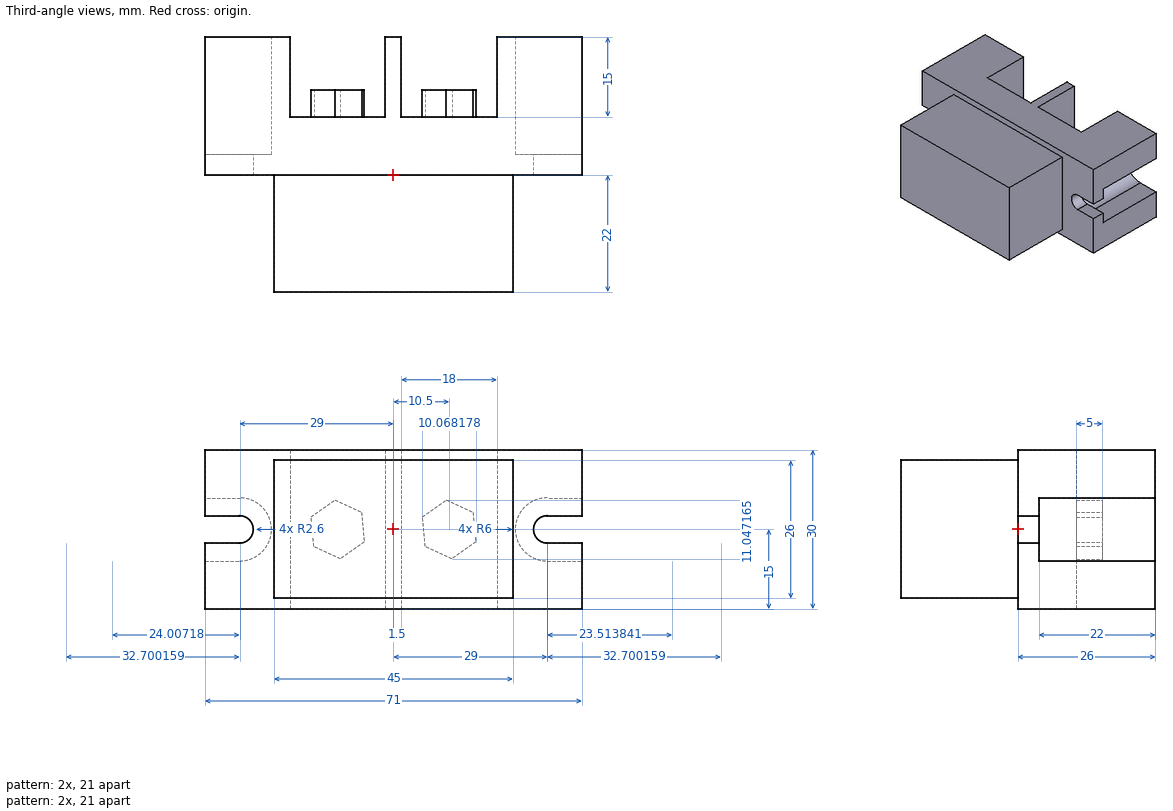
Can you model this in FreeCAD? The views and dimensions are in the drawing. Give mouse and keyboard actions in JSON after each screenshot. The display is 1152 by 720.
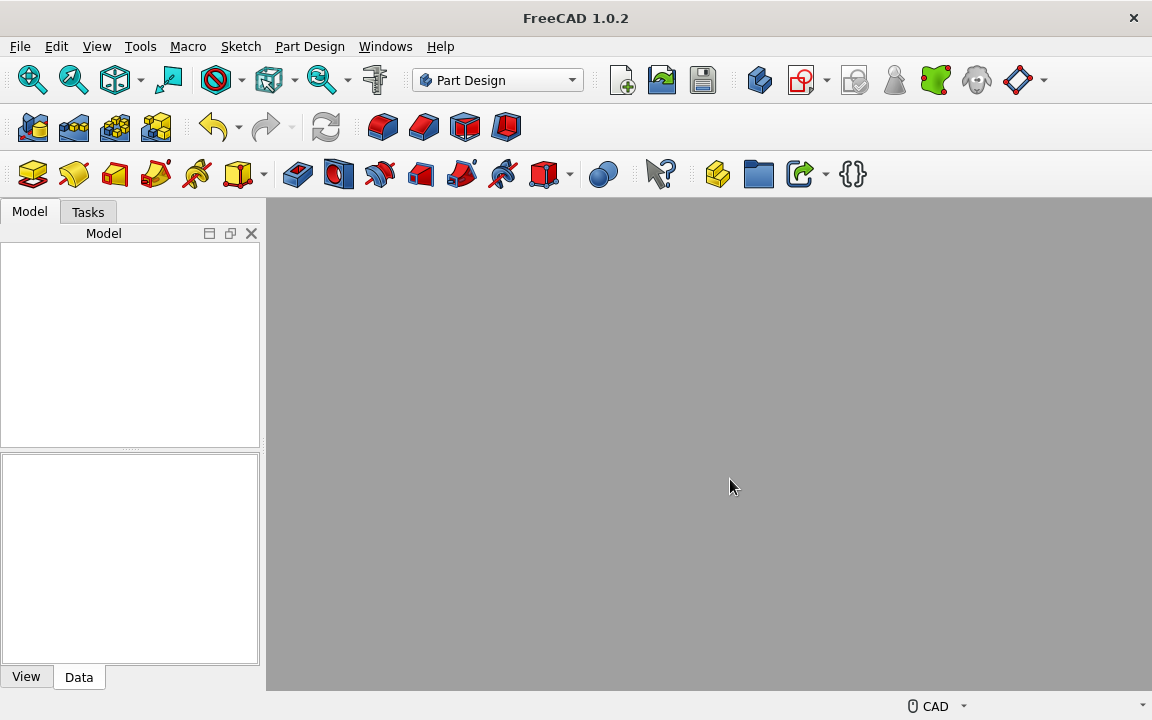
{"action": "left_click", "coordinate": [621, 80]}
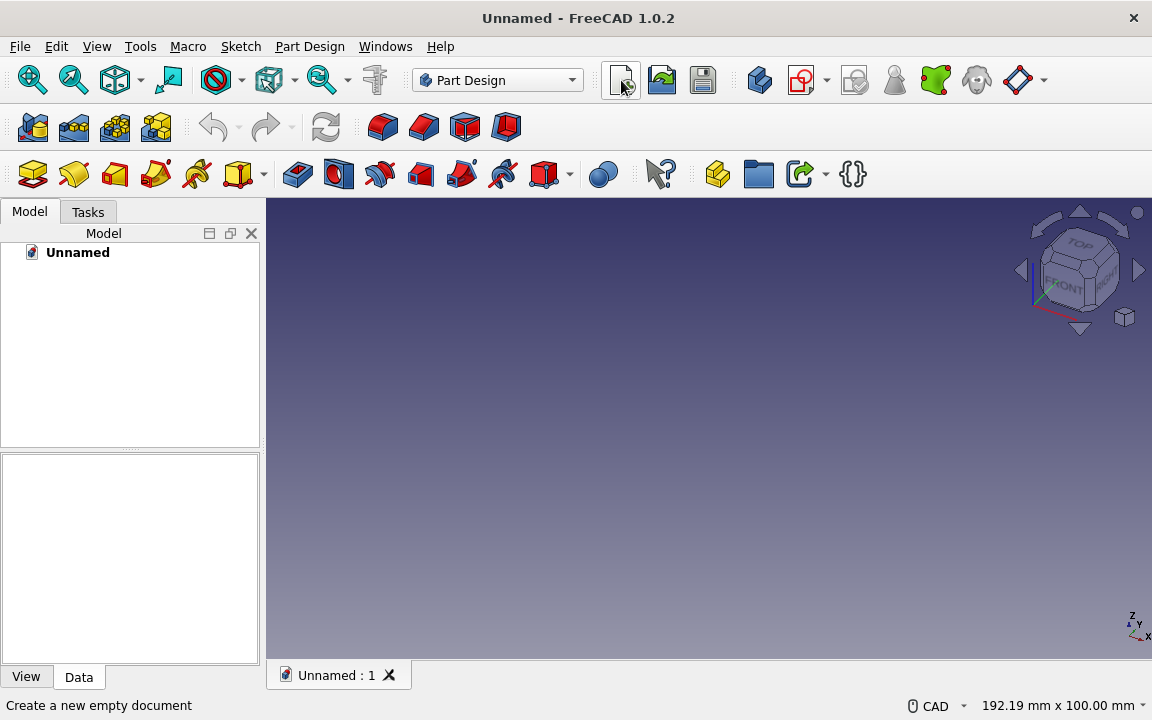
{"action": "left_click", "coordinate": [800, 80]}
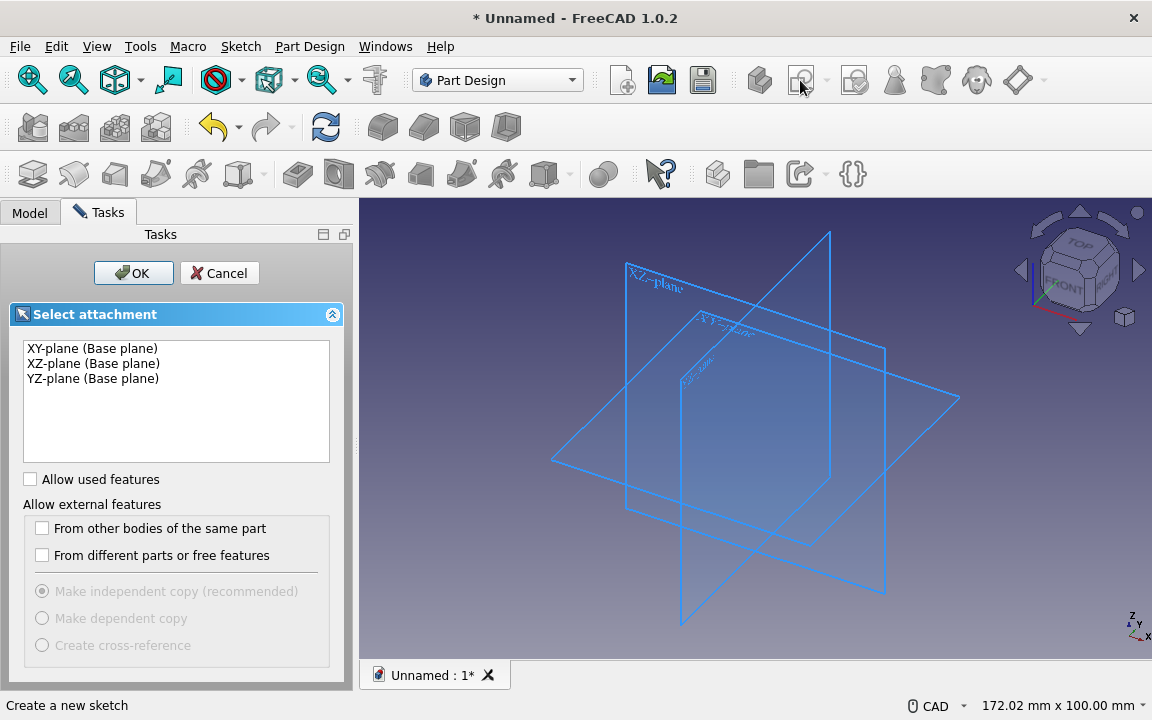
{"action": "left_click", "coordinate": [84, 364]}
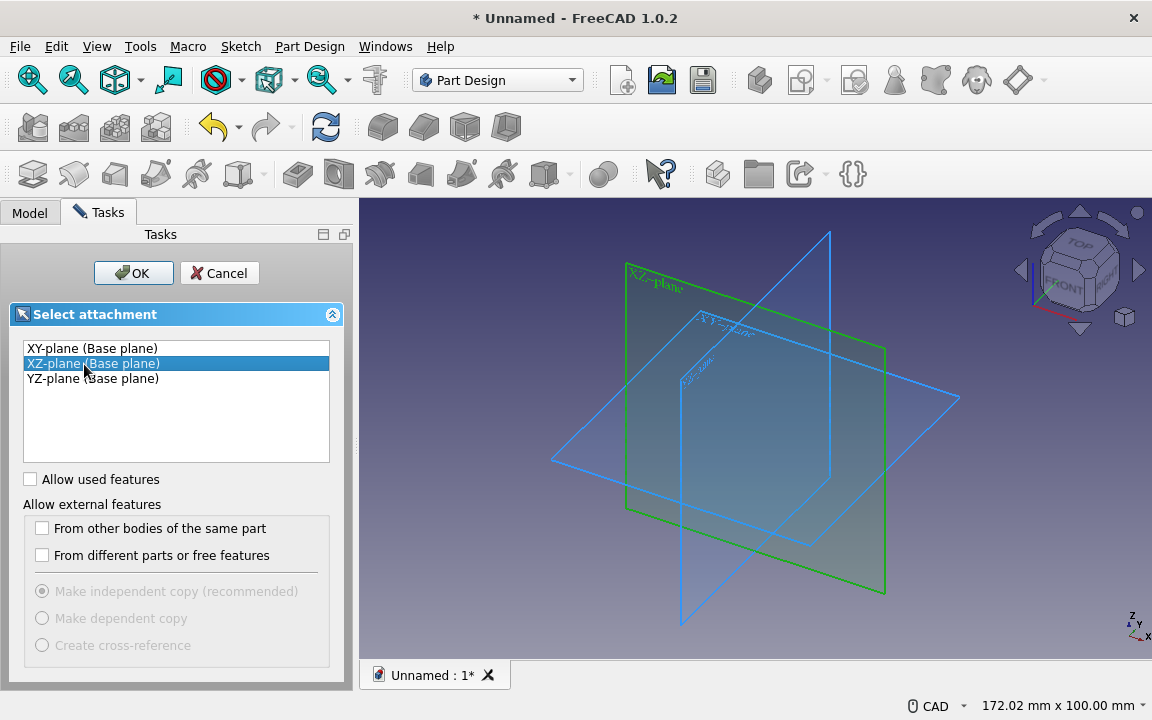
{"action": "left_click", "coordinate": [134, 273]}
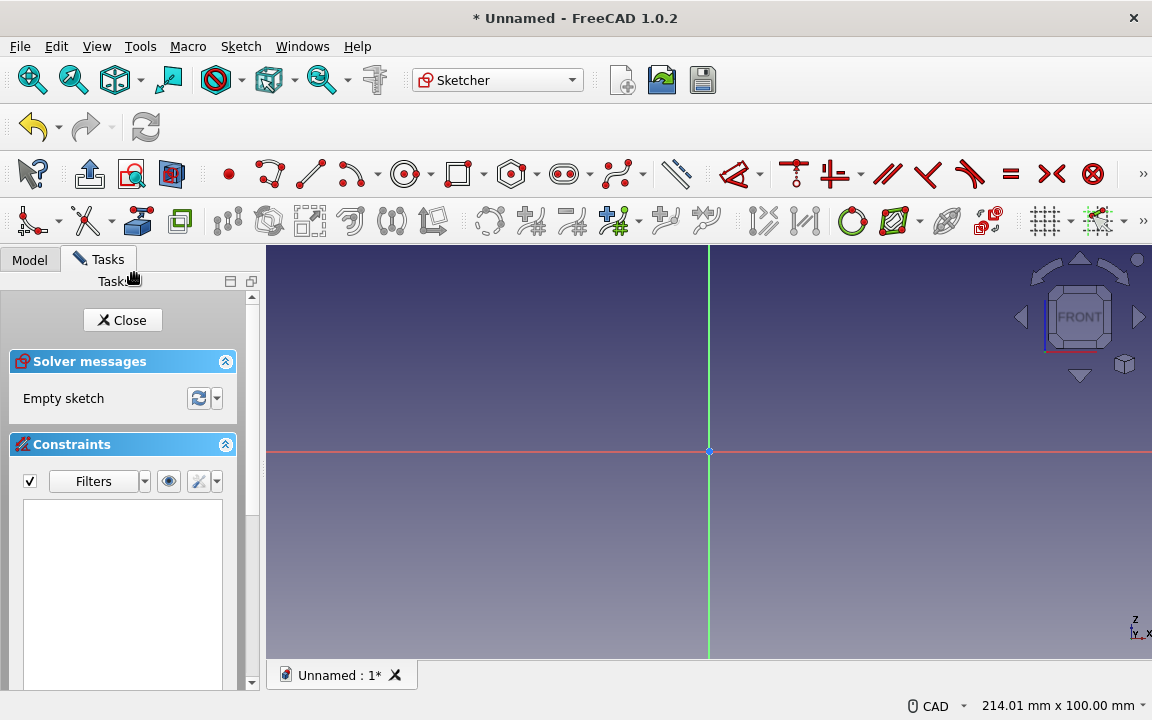
{"action": "scroll", "coordinate": [792, 452], "scroll_direction": "up", "scroll_amount": 3}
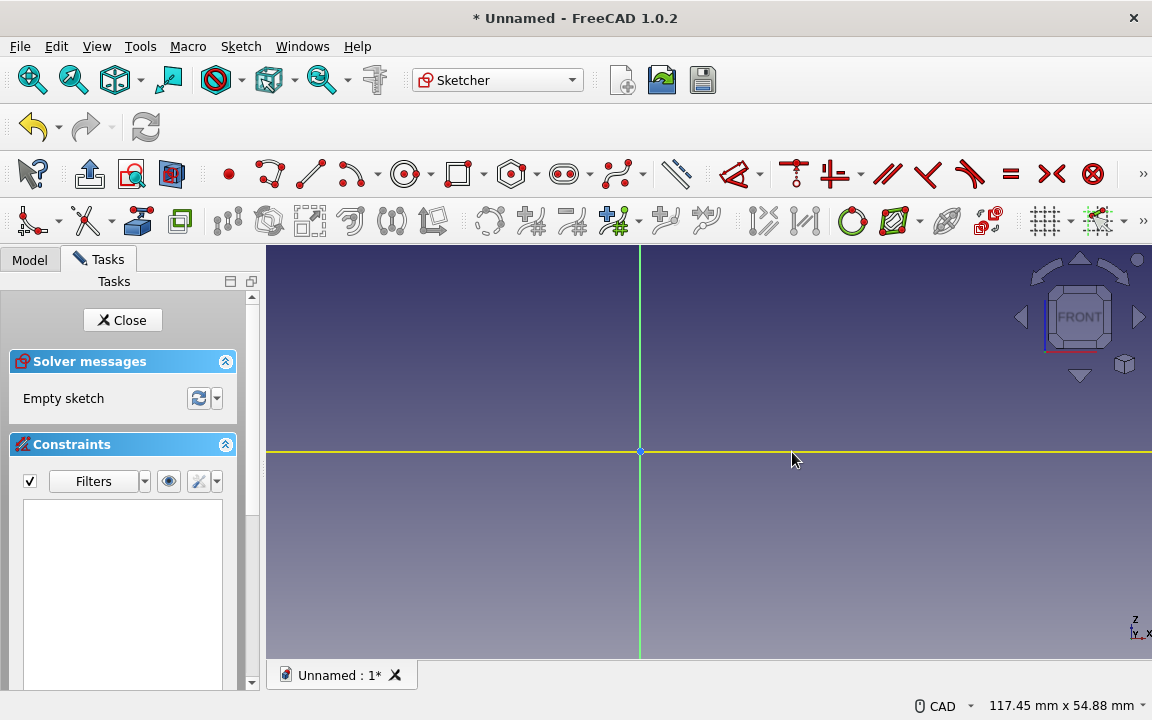
{"action": "key", "text": "g v"}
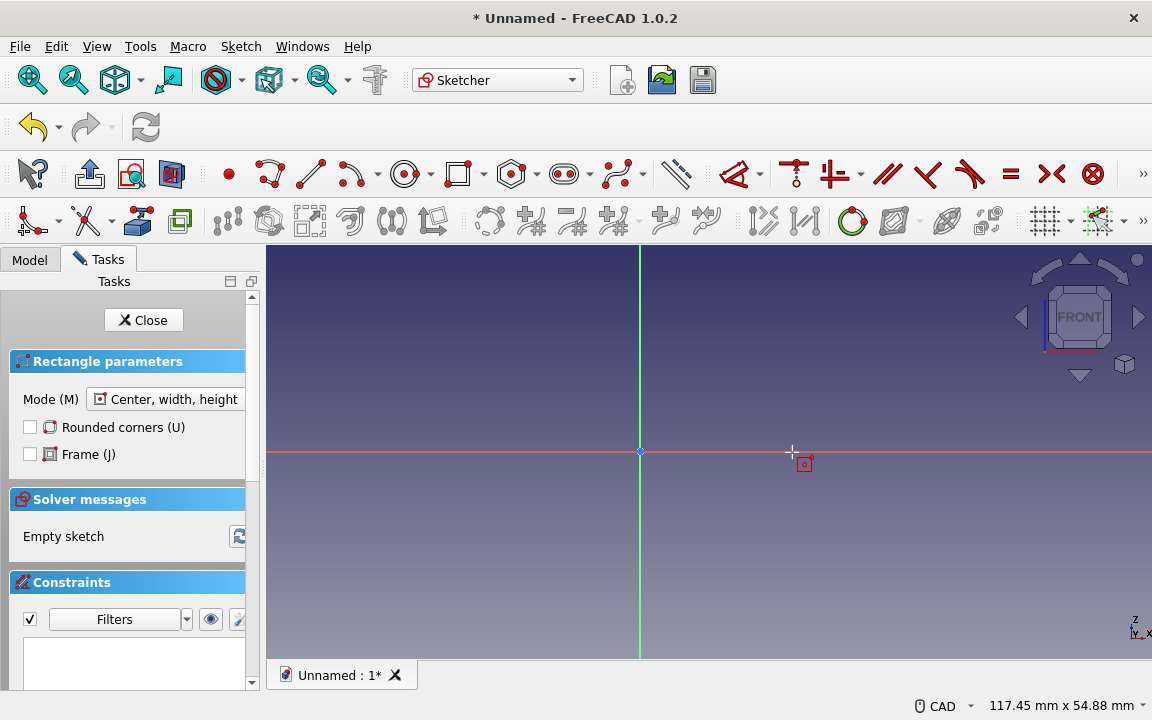
{"action": "left_click", "coordinate": [640, 452]}
{"action": "mouse_move", "coordinate": [908, 338]}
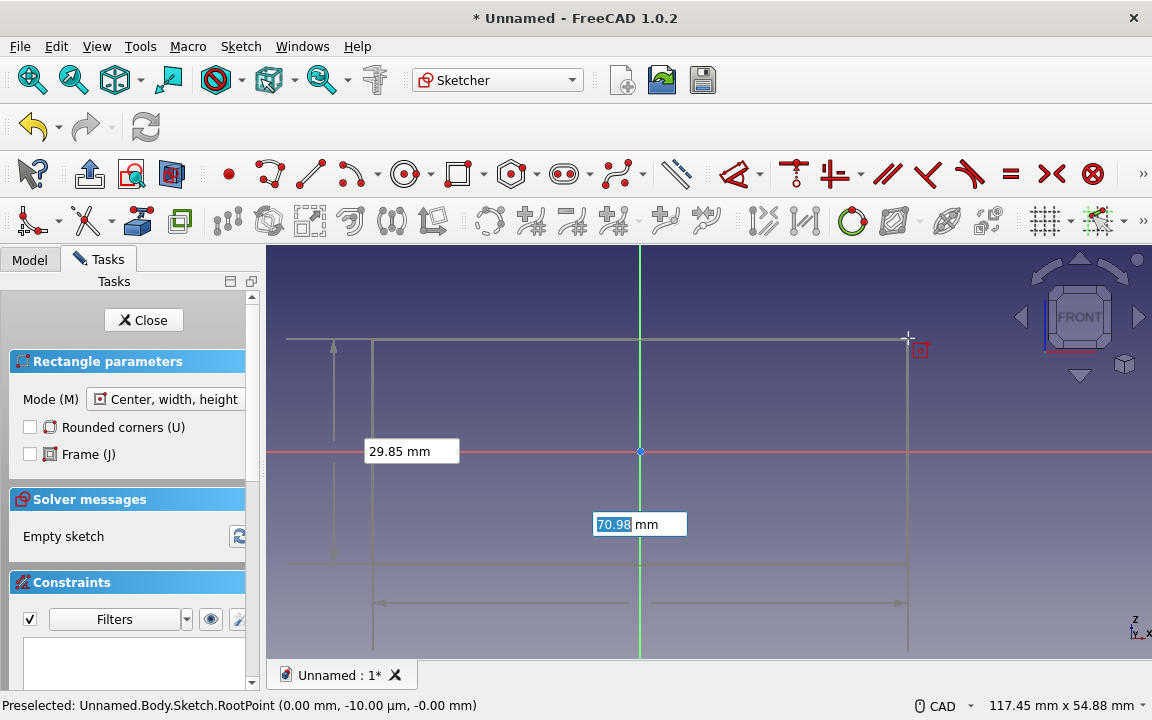
{"action": "type", "text": "71"}
{"action": "key", "text": "Tab"}
{"action": "type", "text": "30"}
{"action": "key", "text": "Return"}
{"action": "key", "text": "Escape"}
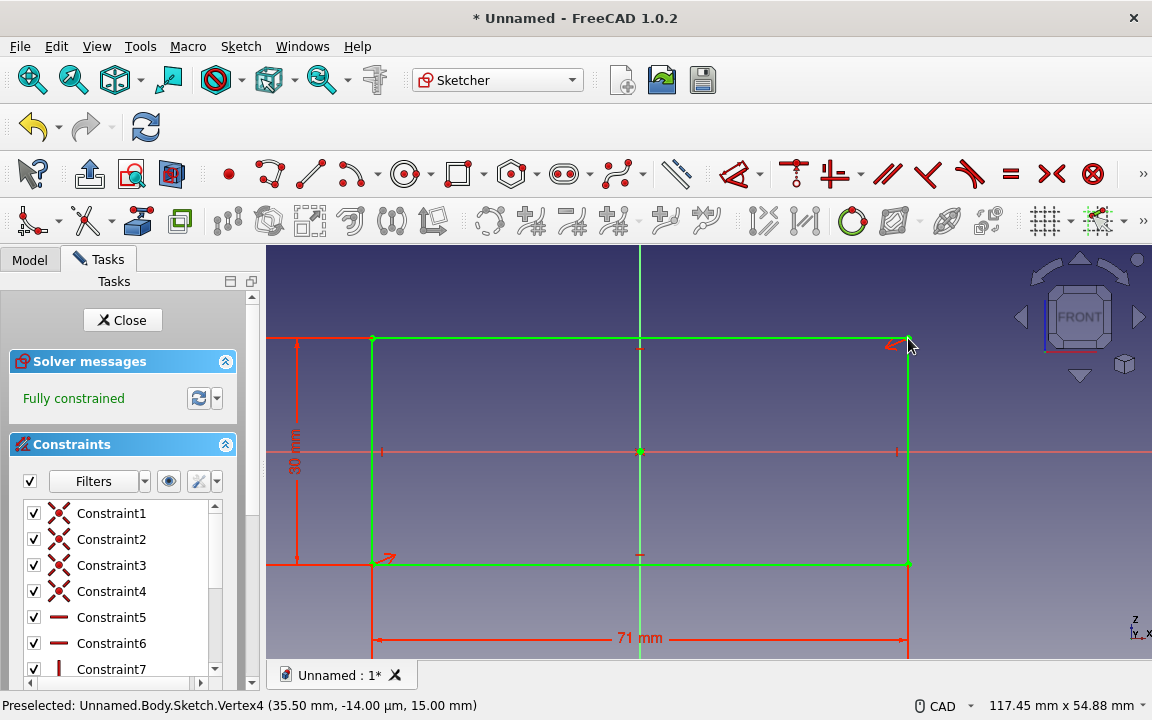
{"action": "left_click", "coordinate": [123, 320]}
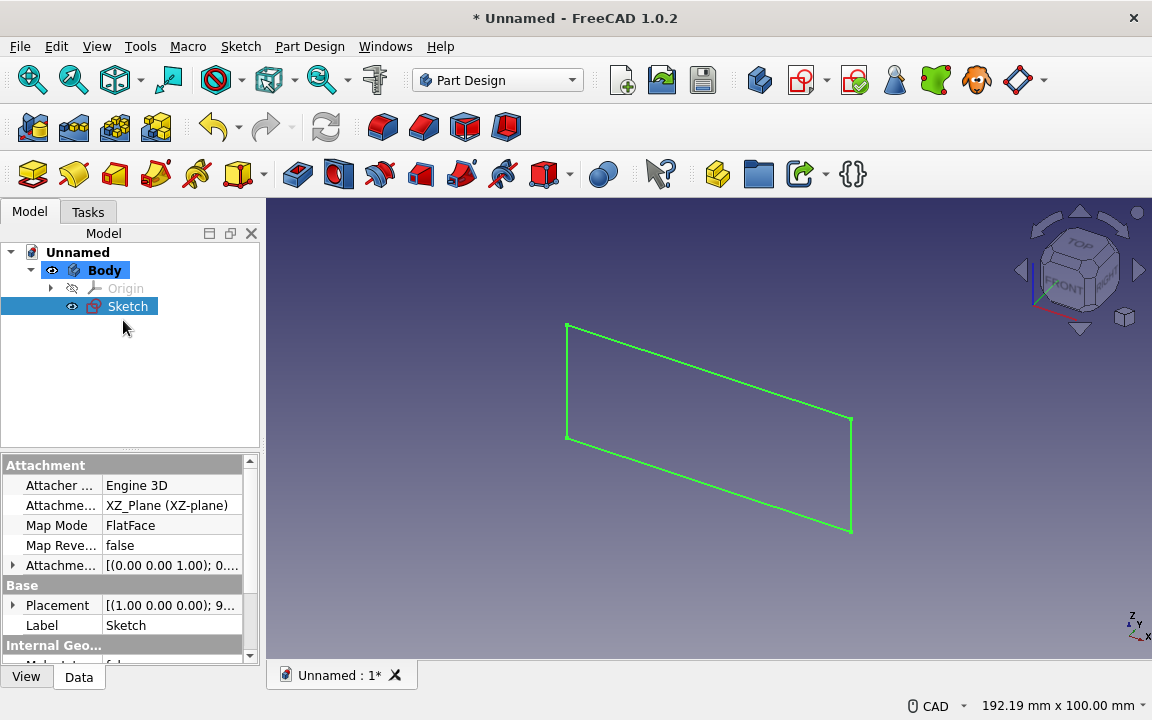
{"action": "left_click", "coordinate": [33, 174]}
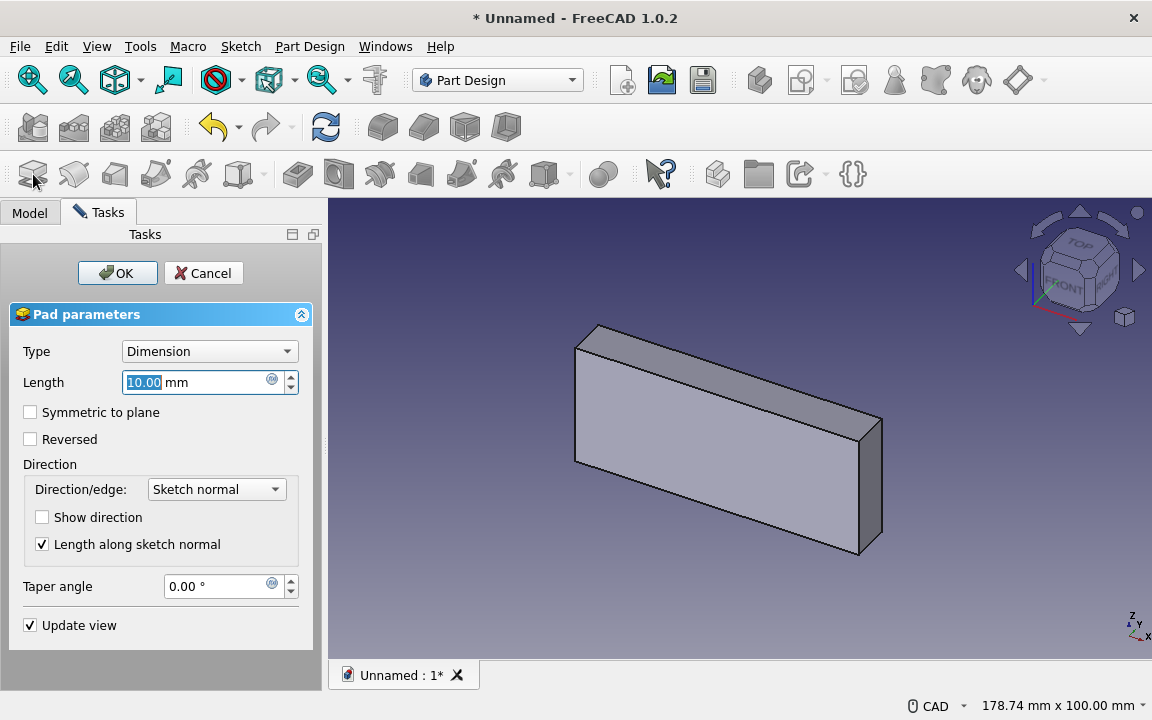
{"action": "type", "text": "26"}
{"action": "key", "text": "Tab"}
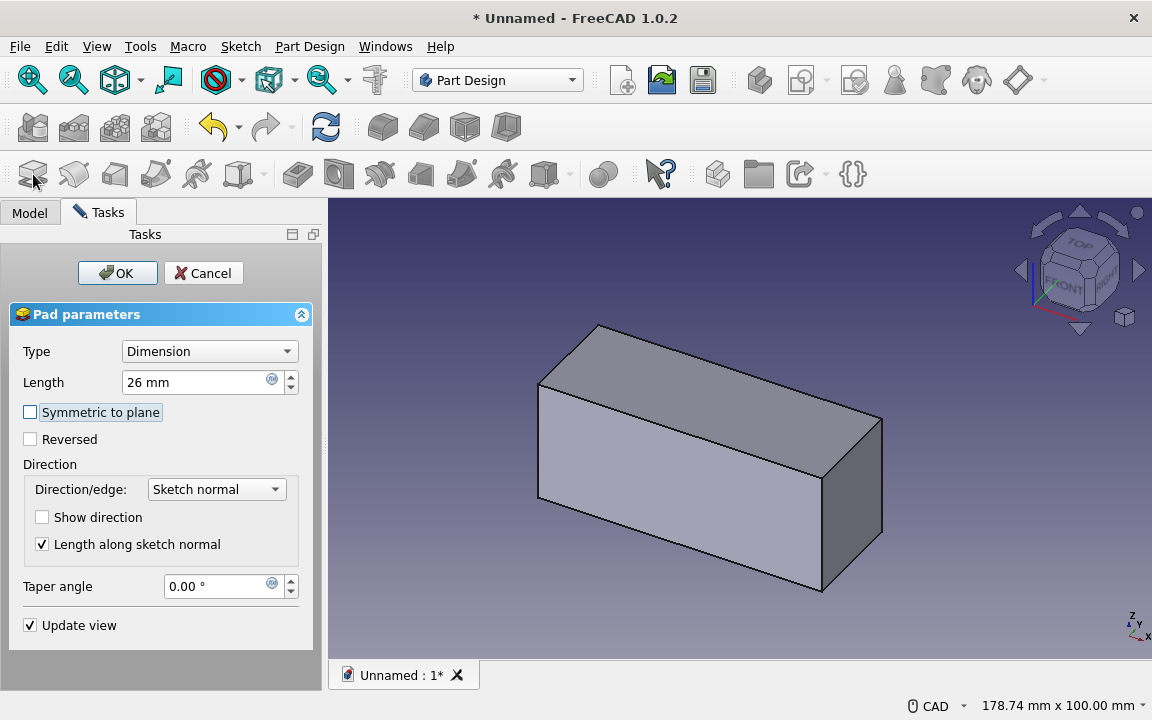
{"action": "left_click", "coordinate": [31, 439]}